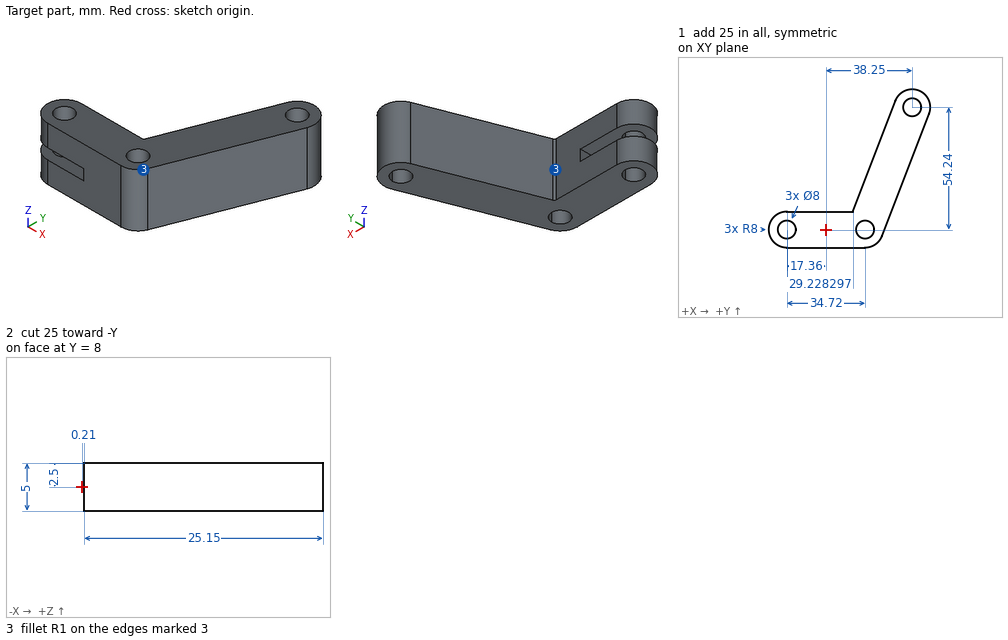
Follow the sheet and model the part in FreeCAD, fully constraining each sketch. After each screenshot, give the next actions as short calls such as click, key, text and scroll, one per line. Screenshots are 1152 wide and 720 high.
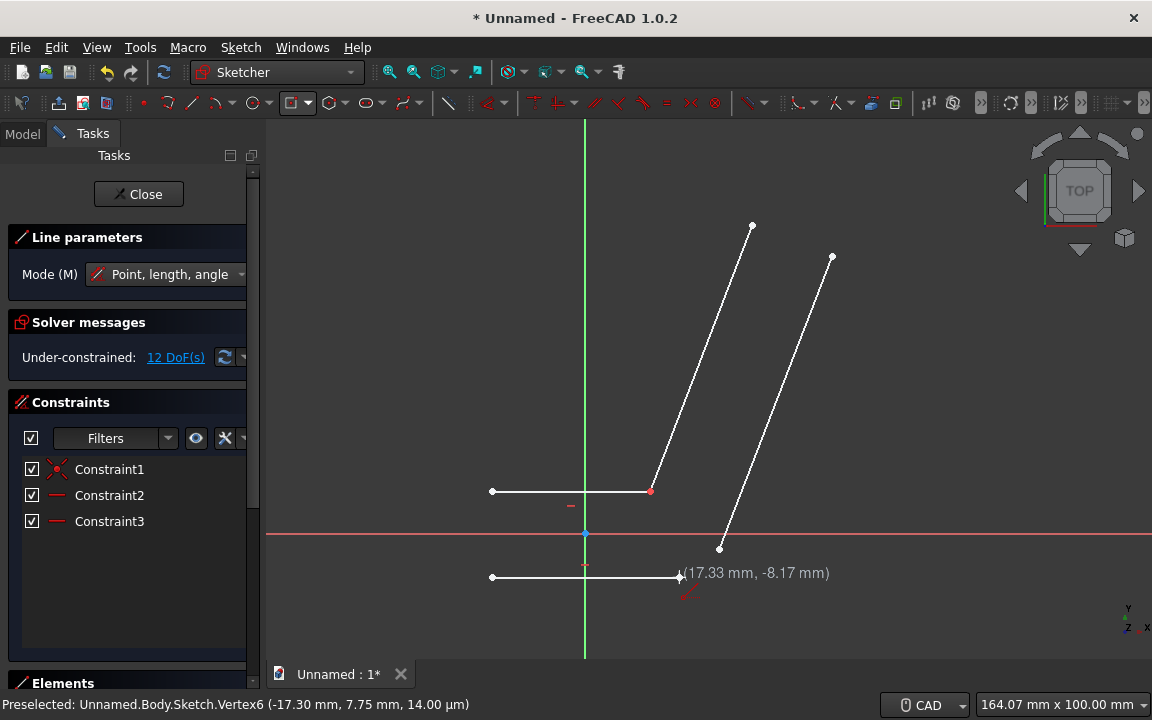
key(g)
key(3)
key(a)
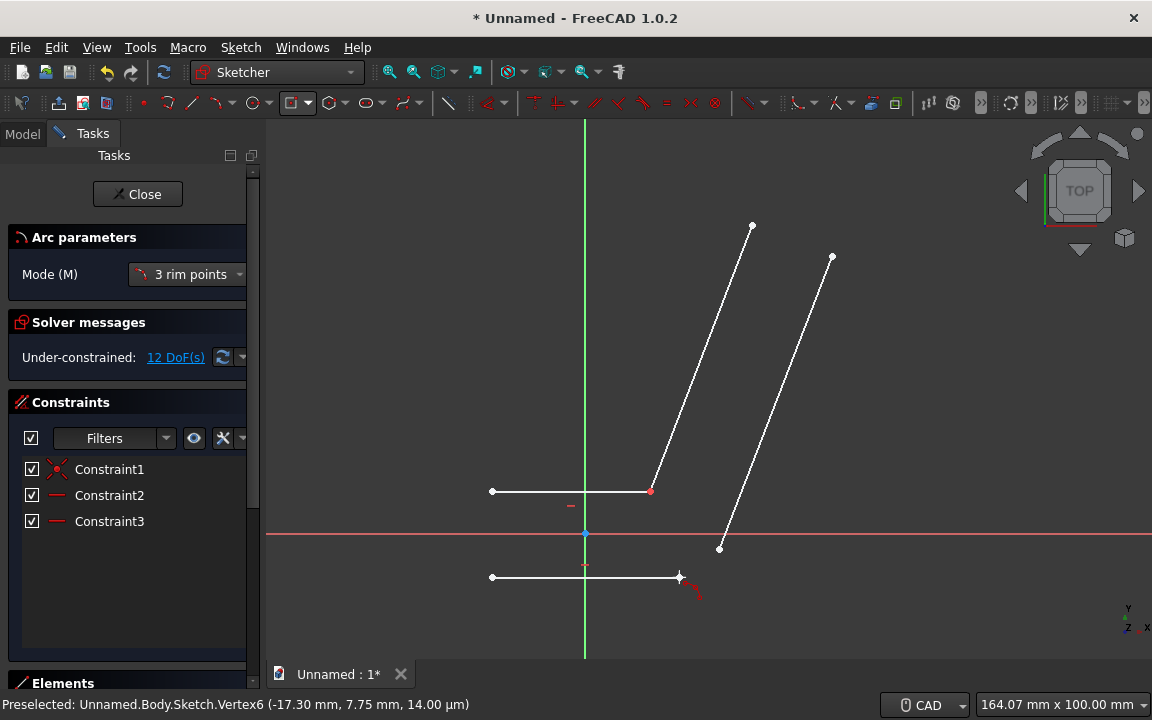
click(832, 257)
click(752, 226)
click(807, 201)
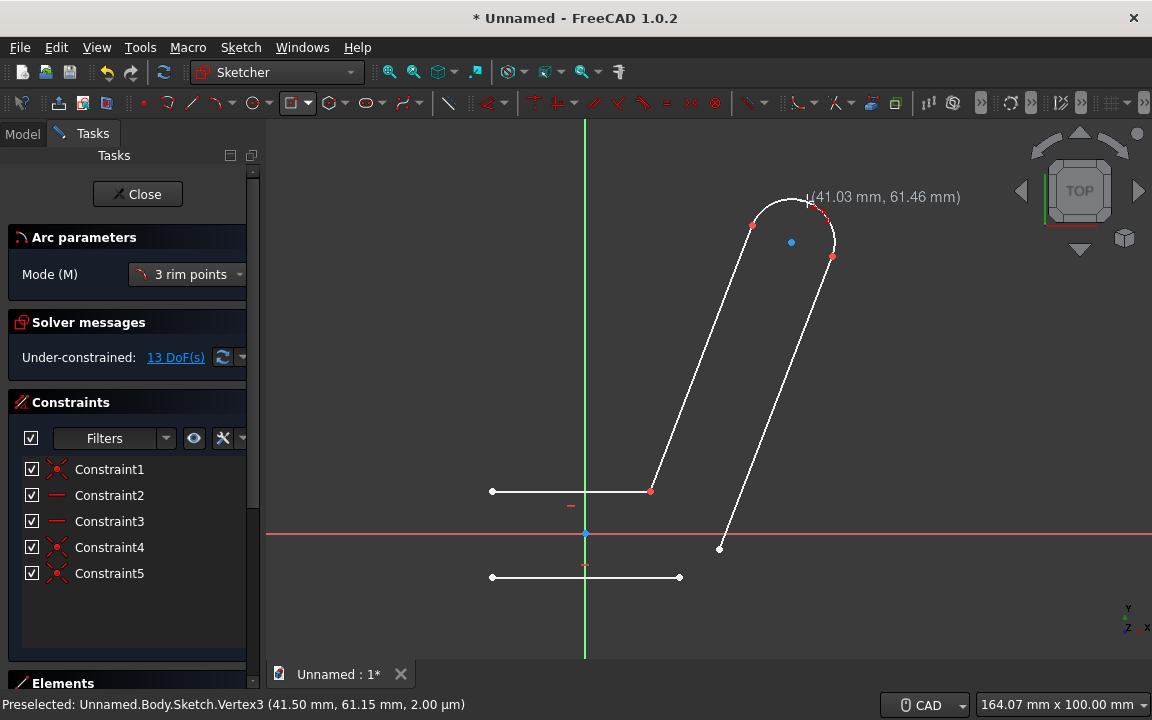
click(492, 492)
click(492, 578)
click(457, 508)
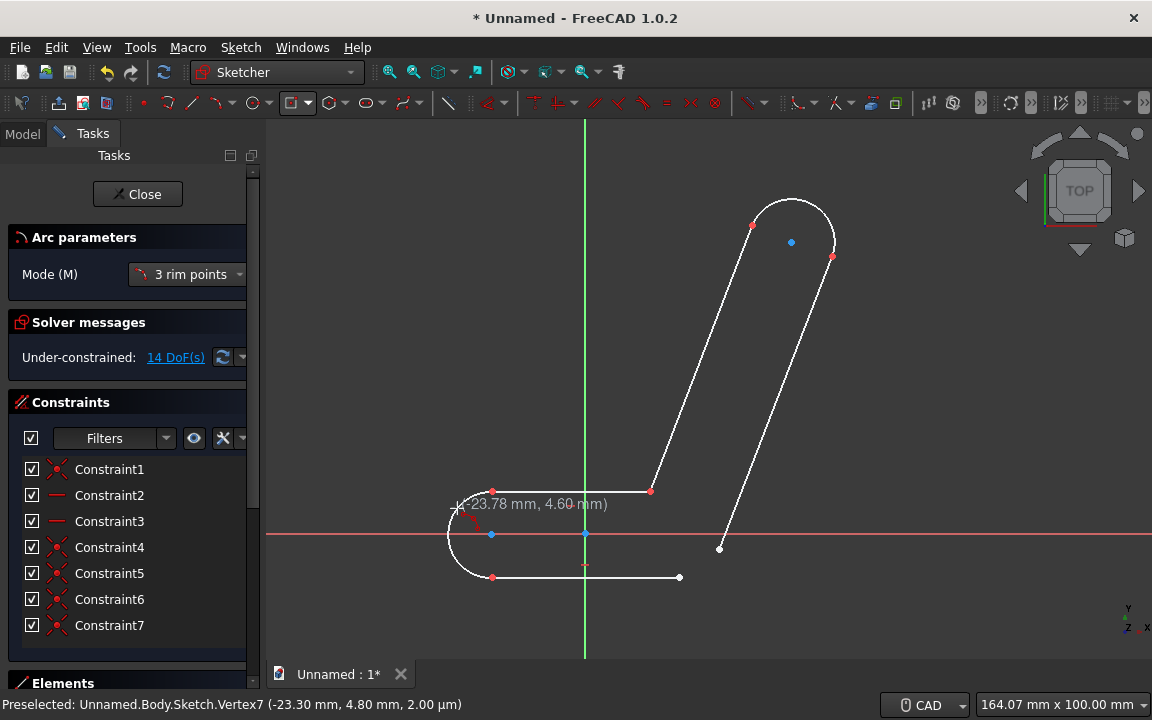
click(679, 578)
click(719, 550)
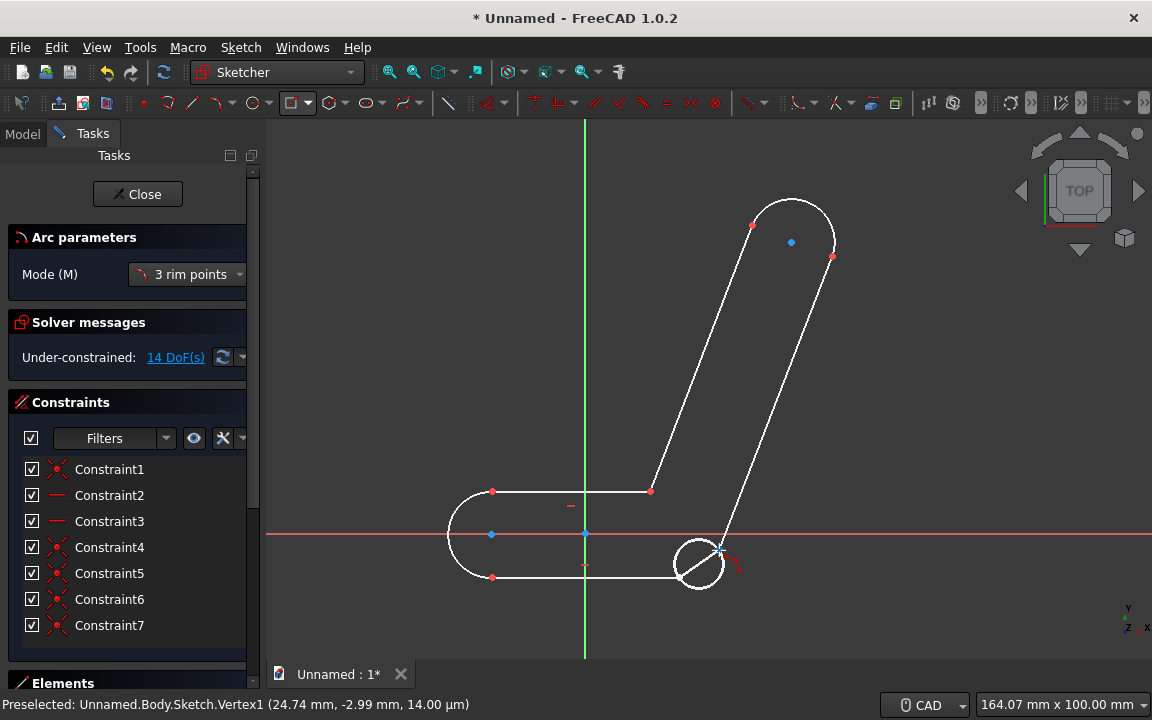
scroll(704, 569, up, 4)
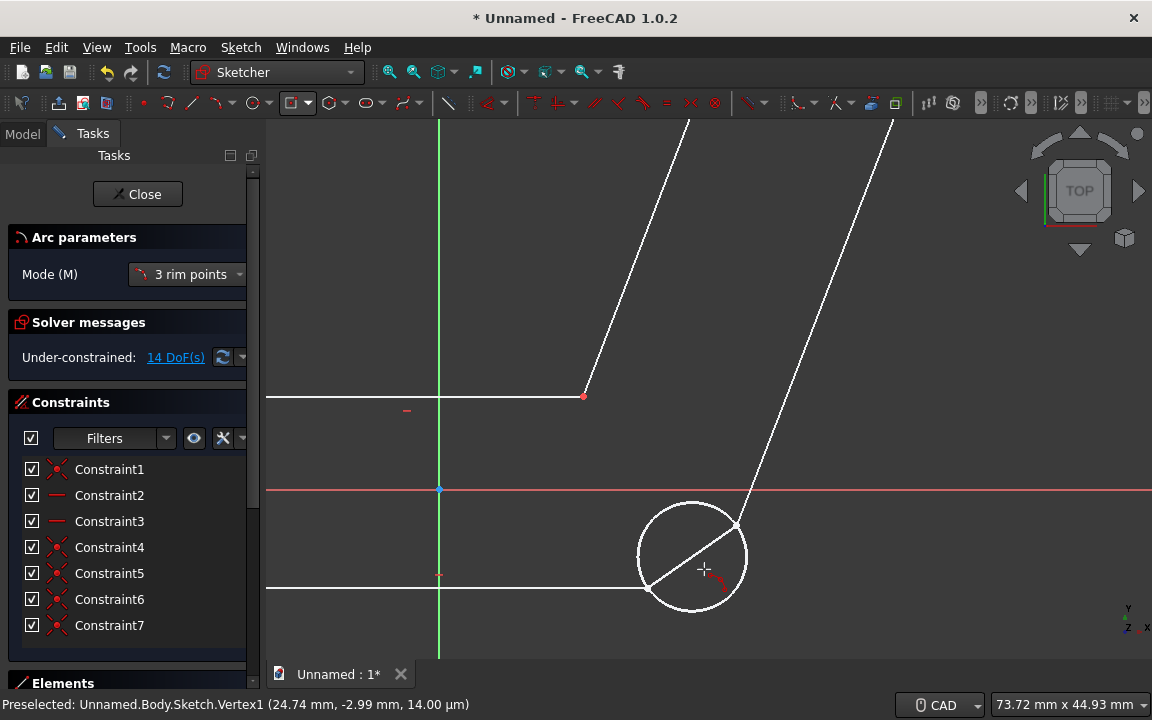
click(703, 569)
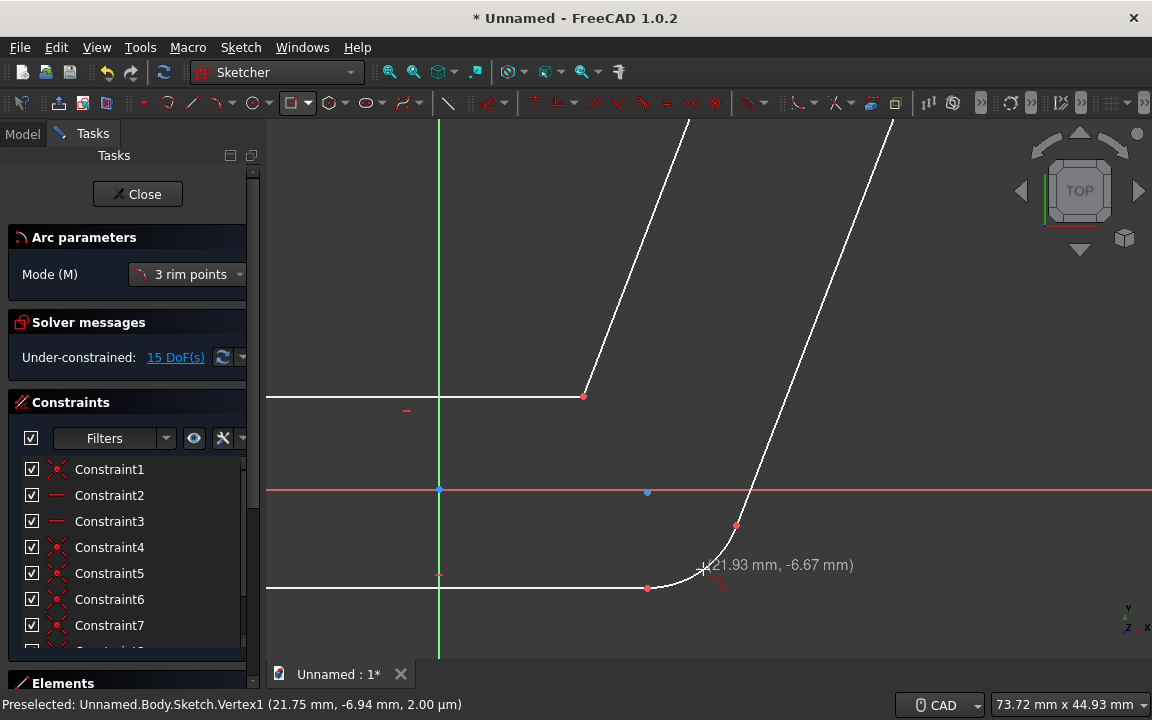
click(254, 104)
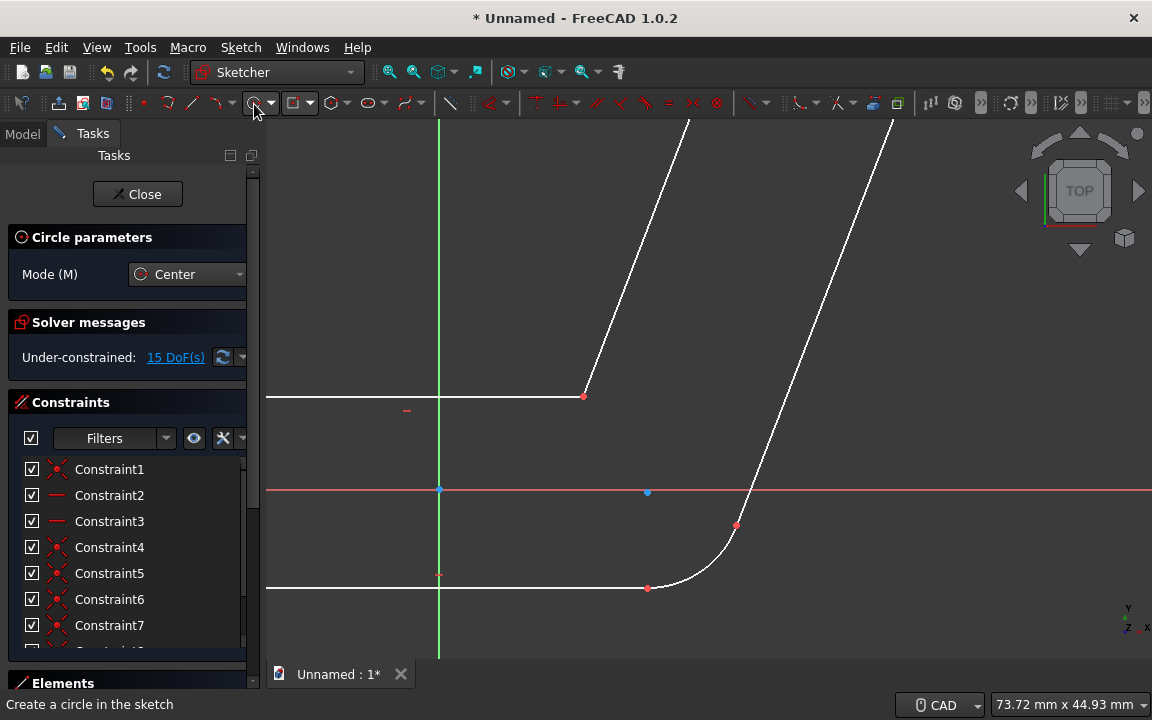
scroll(705, 570, down, 4)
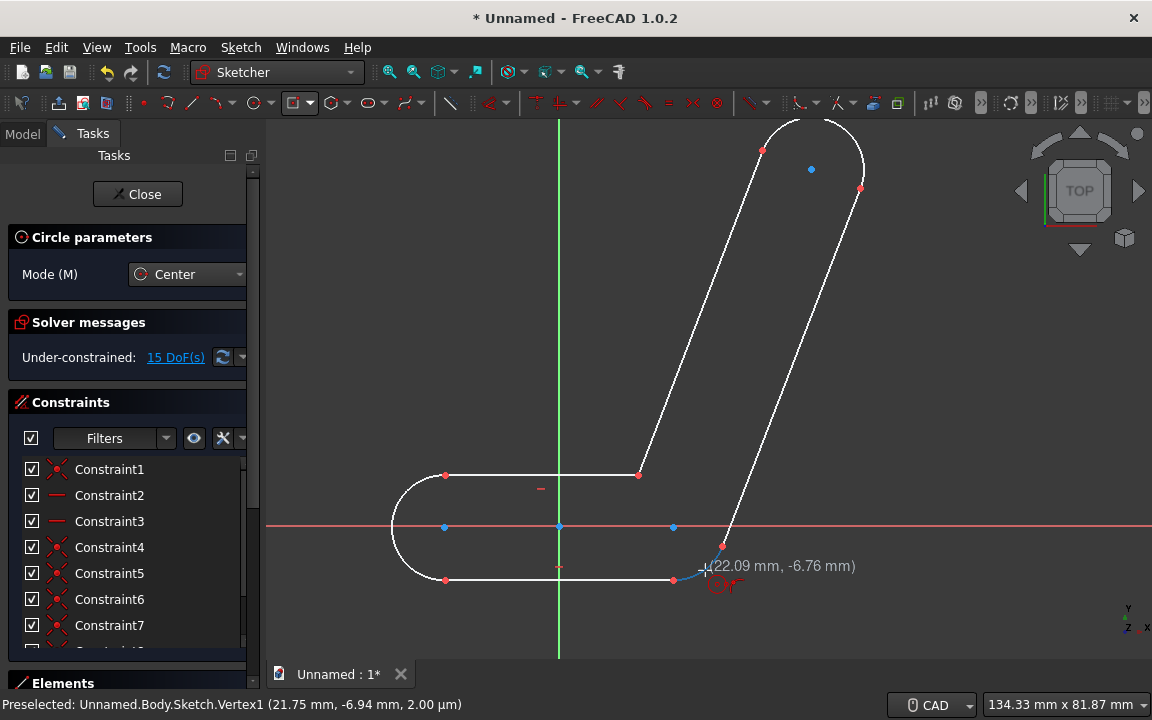
click(492, 534)
click(507, 519)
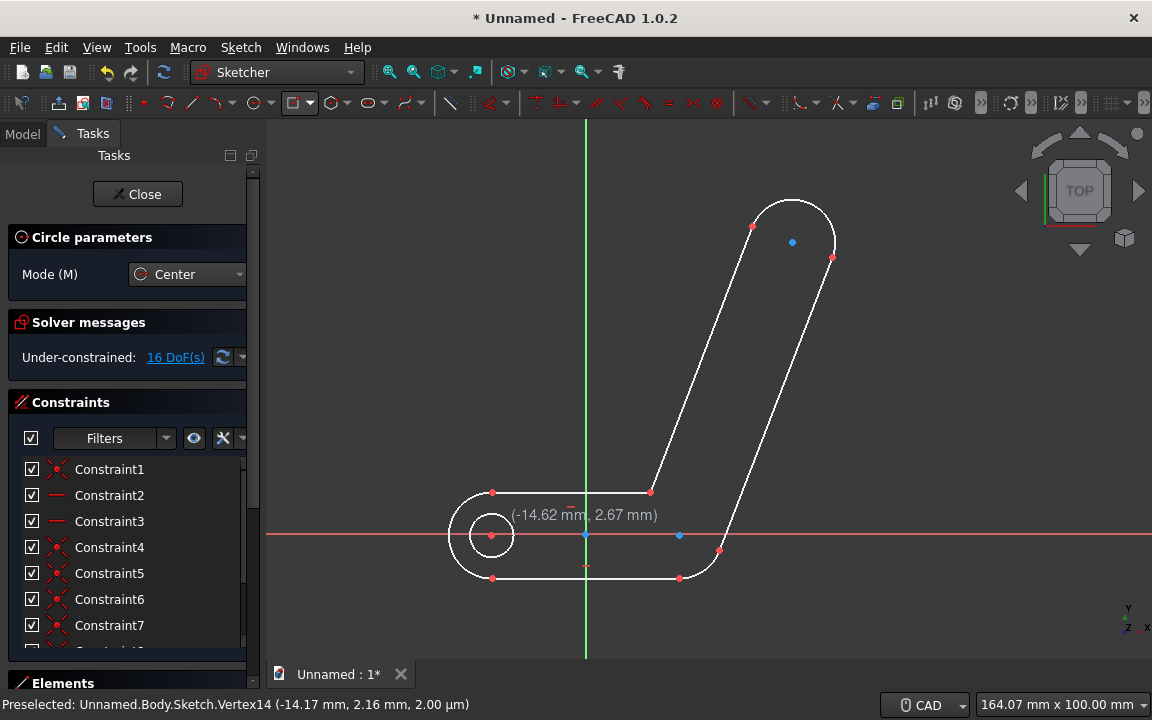
click(680, 534)
click(695, 519)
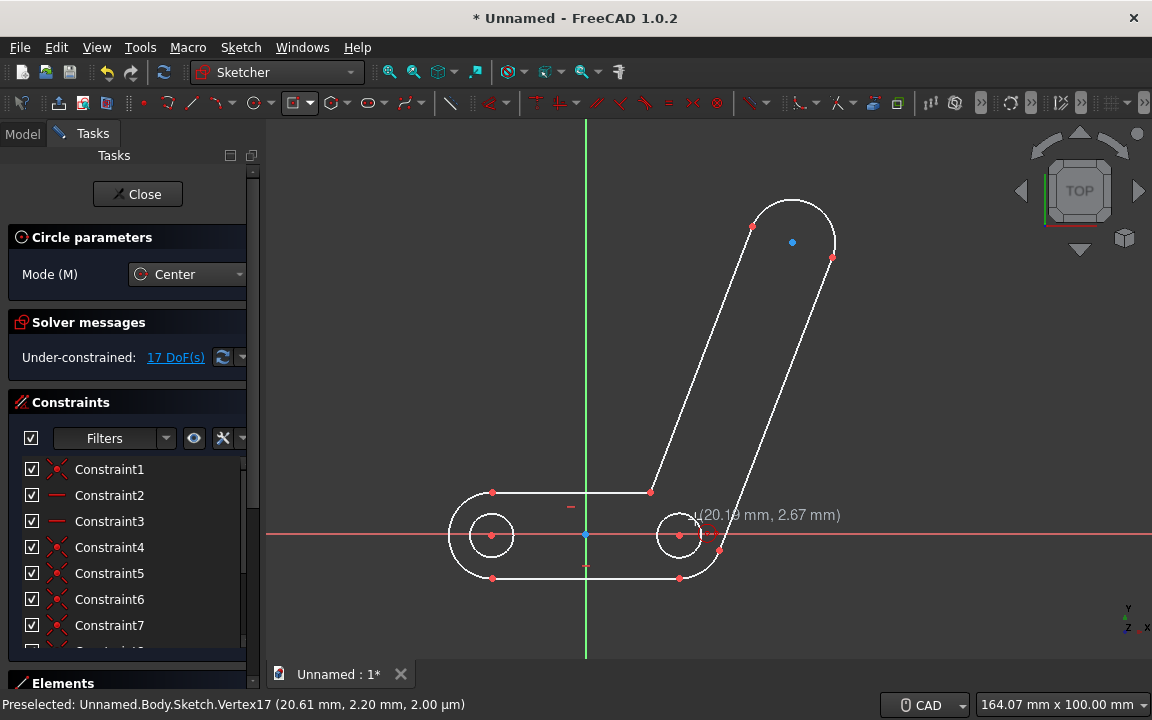
click(793, 242)
click(808, 226)
key(Escape)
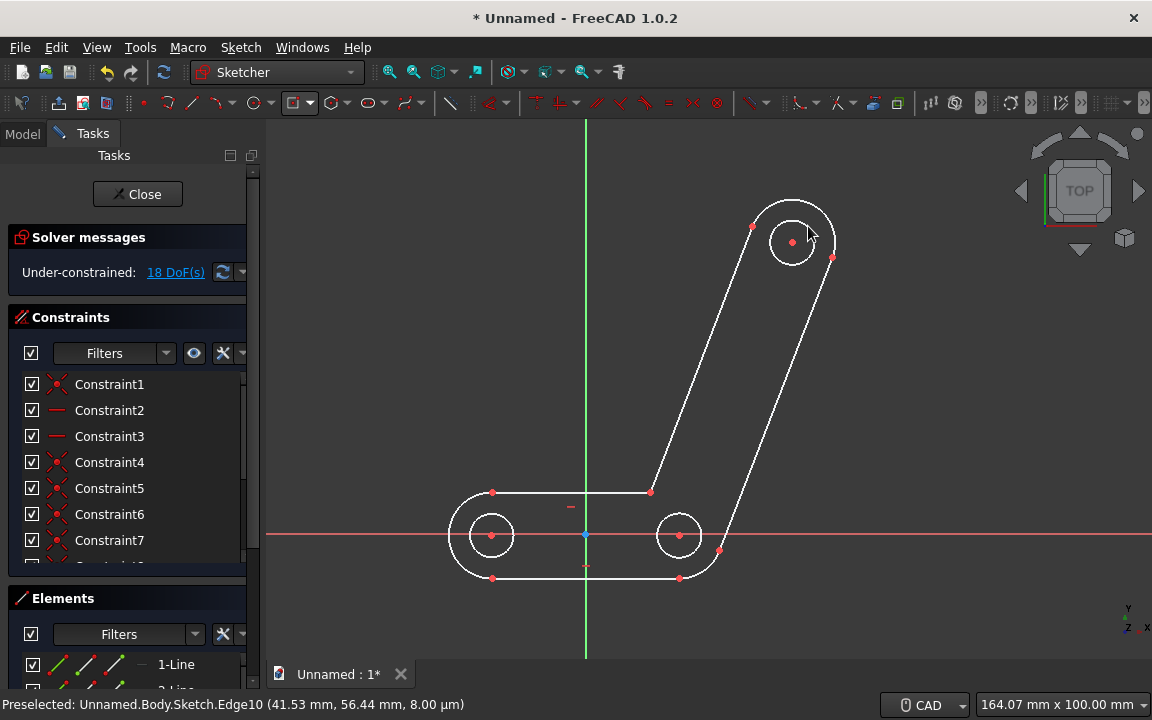
click(753, 463)